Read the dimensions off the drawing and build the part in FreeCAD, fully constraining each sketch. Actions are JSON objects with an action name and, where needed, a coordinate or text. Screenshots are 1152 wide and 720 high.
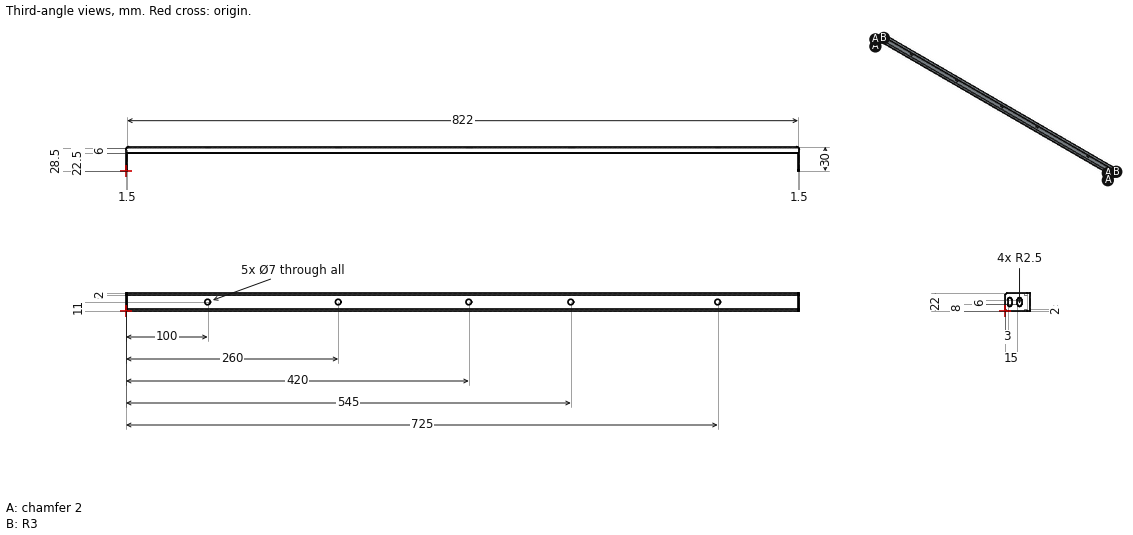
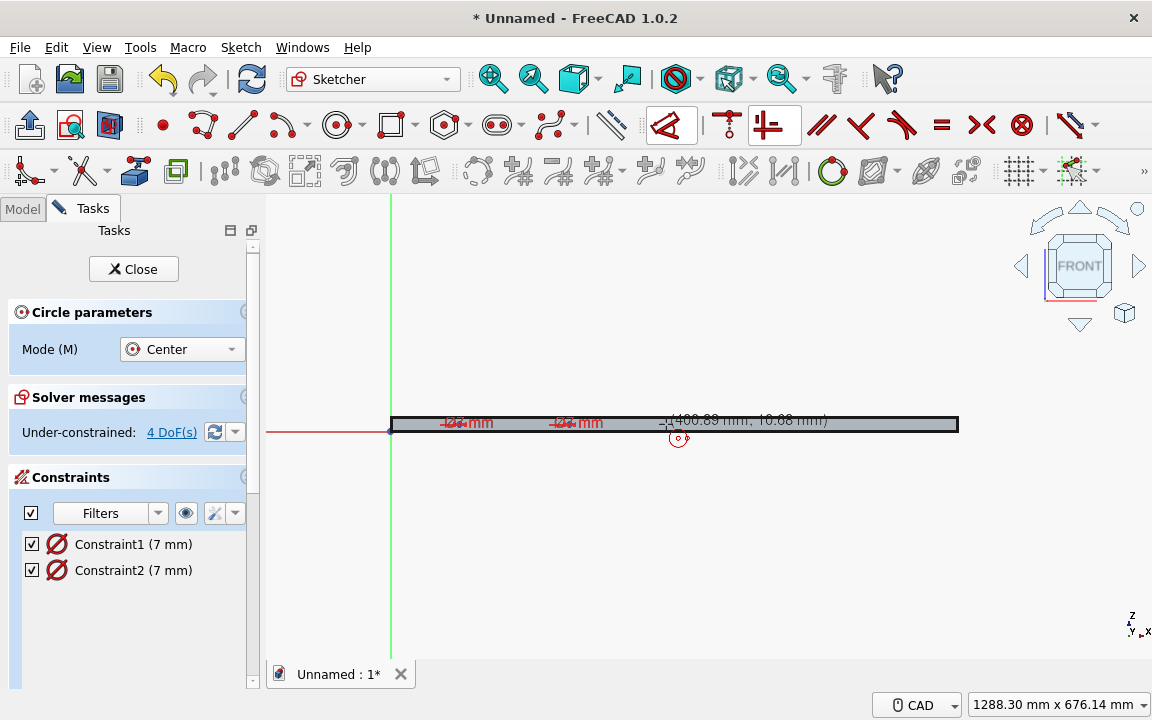
{"action": "scroll", "coordinate": [680, 424], "scroll_direction": "up", "scroll_amount": 4}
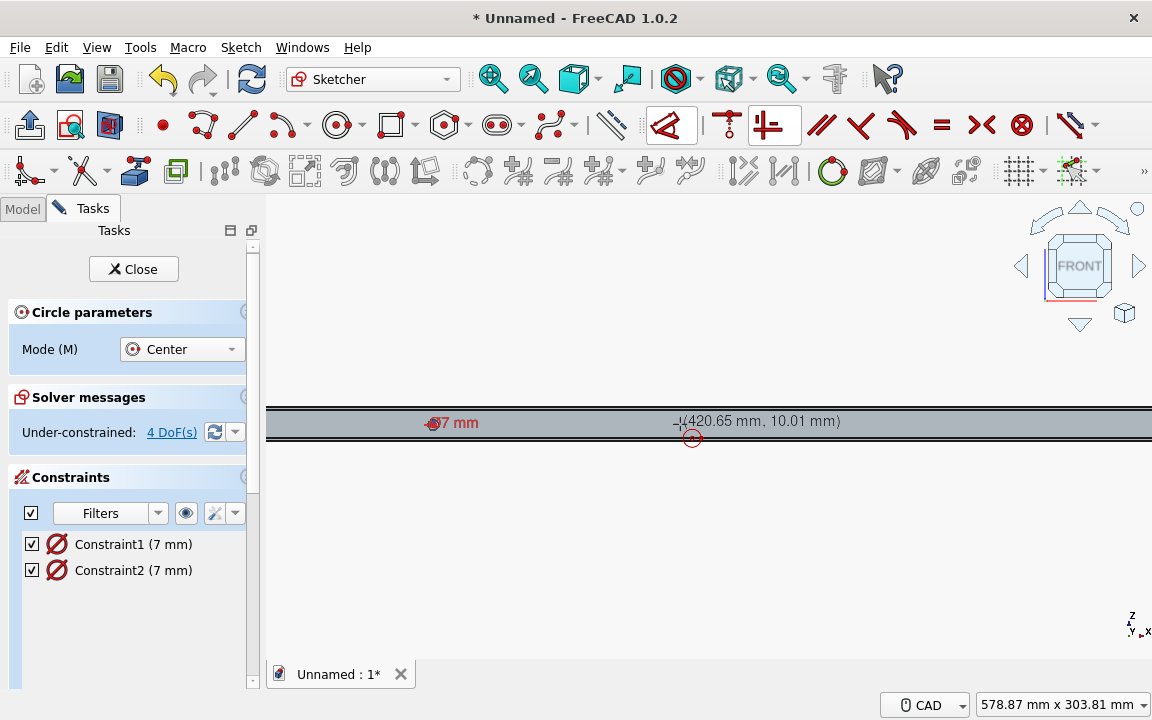
{"action": "left_click", "coordinate": [678, 424]}
{"action": "mouse_move", "coordinate": [682, 420]}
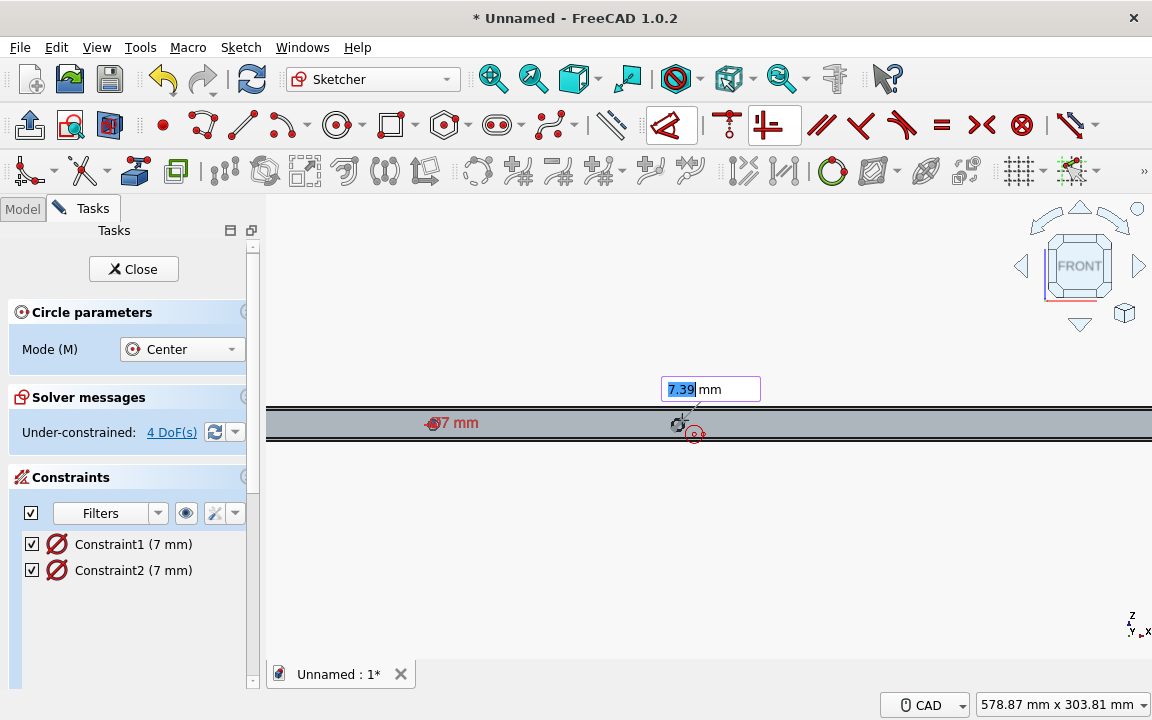
{"action": "type", "text": "7"}
{"action": "key", "text": "Return"}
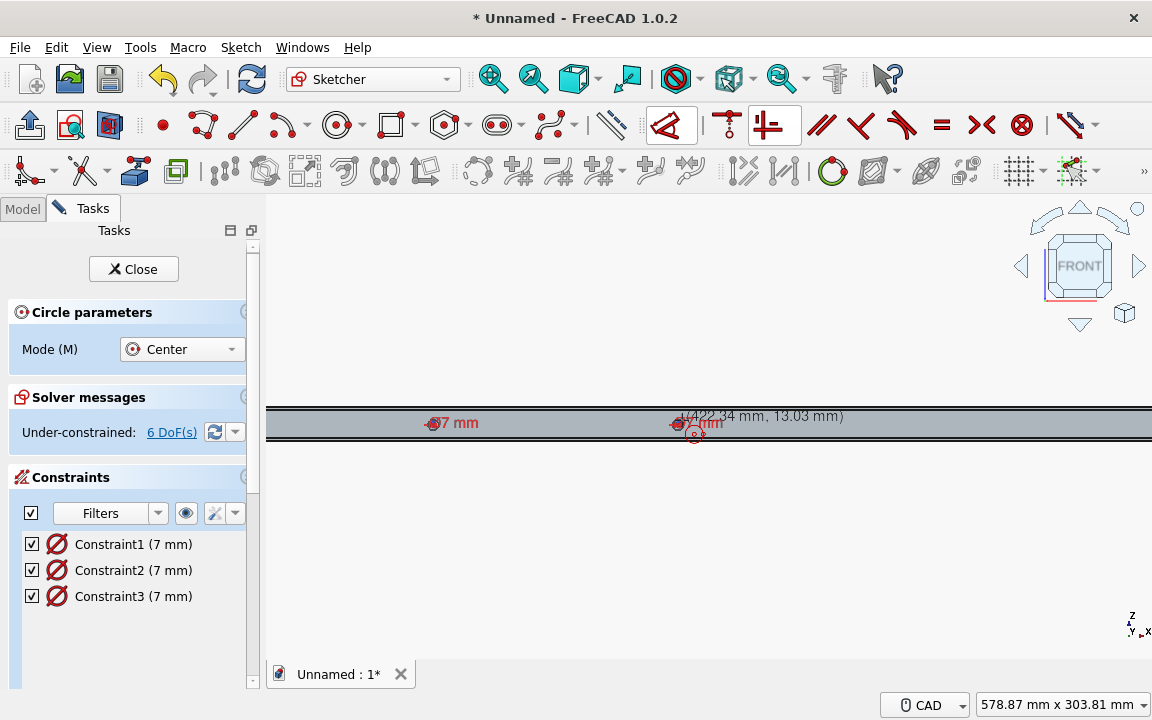
{"action": "scroll", "coordinate": [870, 424], "scroll_direction": "up", "scroll_amount": 8}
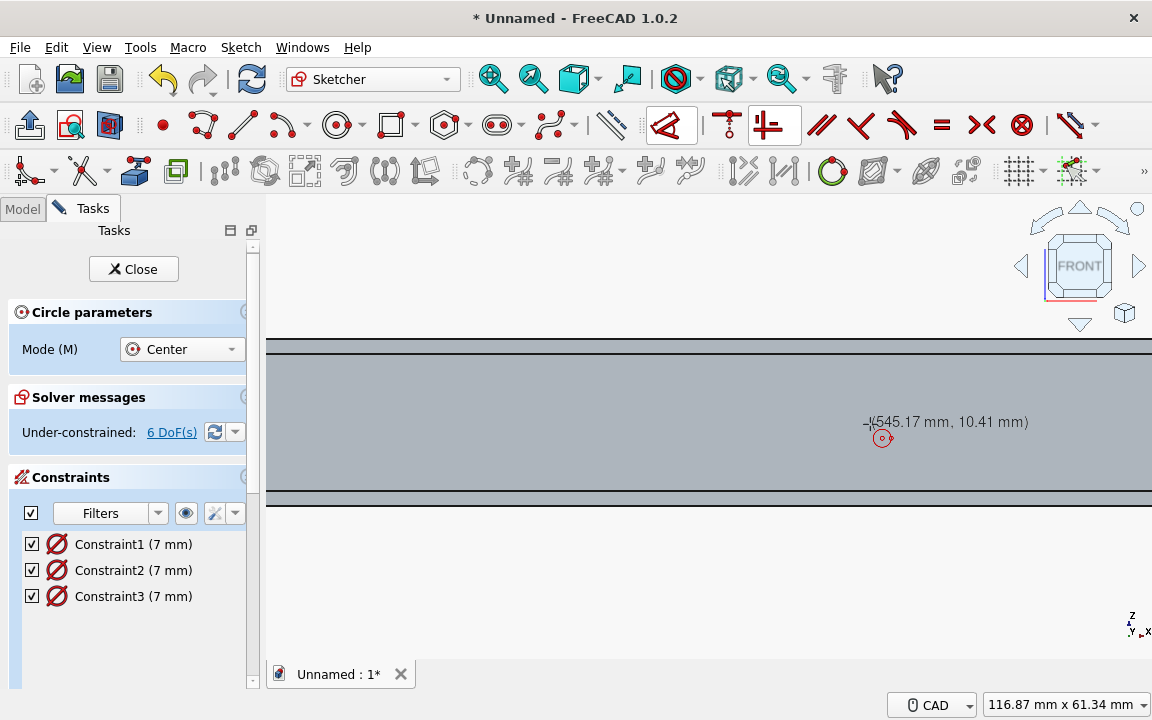
{"action": "scroll", "coordinate": [755, 424], "scroll_direction": "down", "scroll_amount": 12}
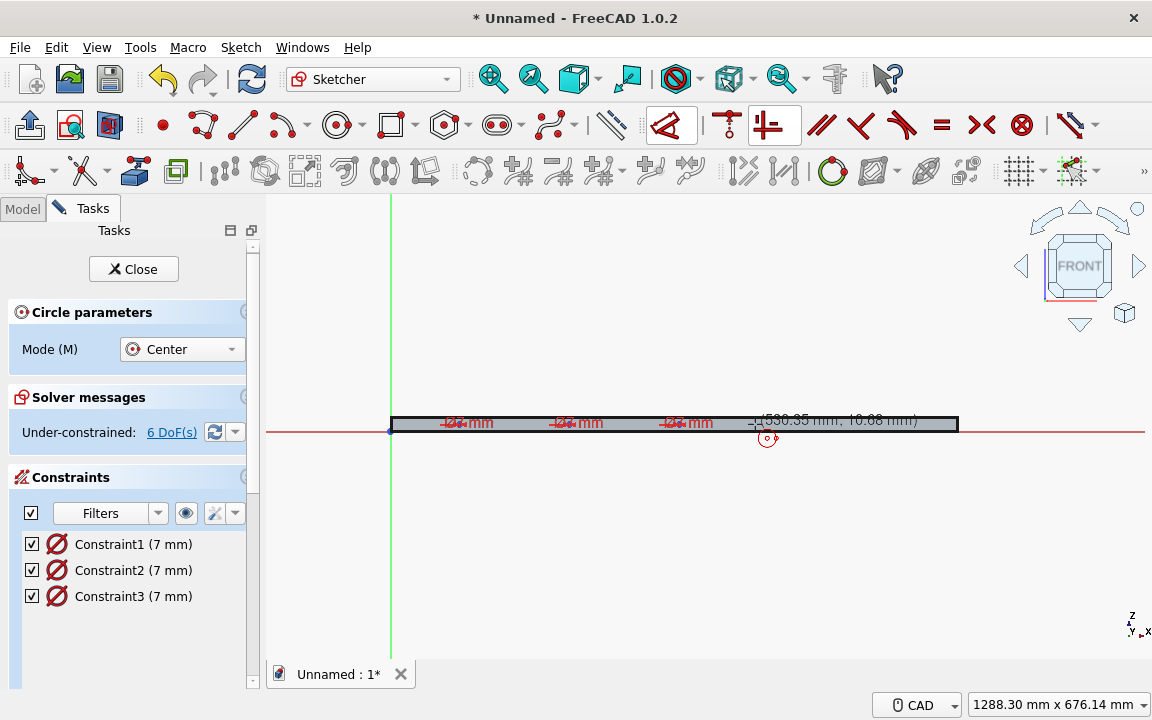
{"action": "scroll", "coordinate": [766, 424], "scroll_direction": "up", "scroll_amount": 4}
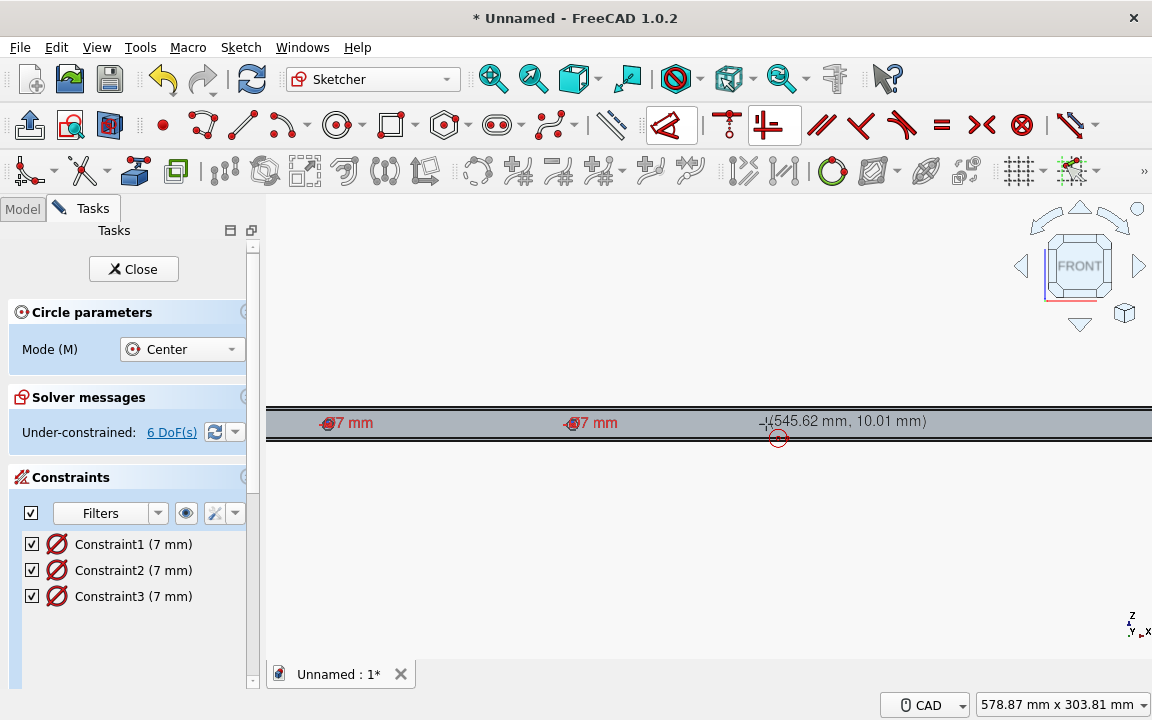
{"action": "left_click", "coordinate": [764, 424]}
{"action": "mouse_move", "coordinate": [768, 420]}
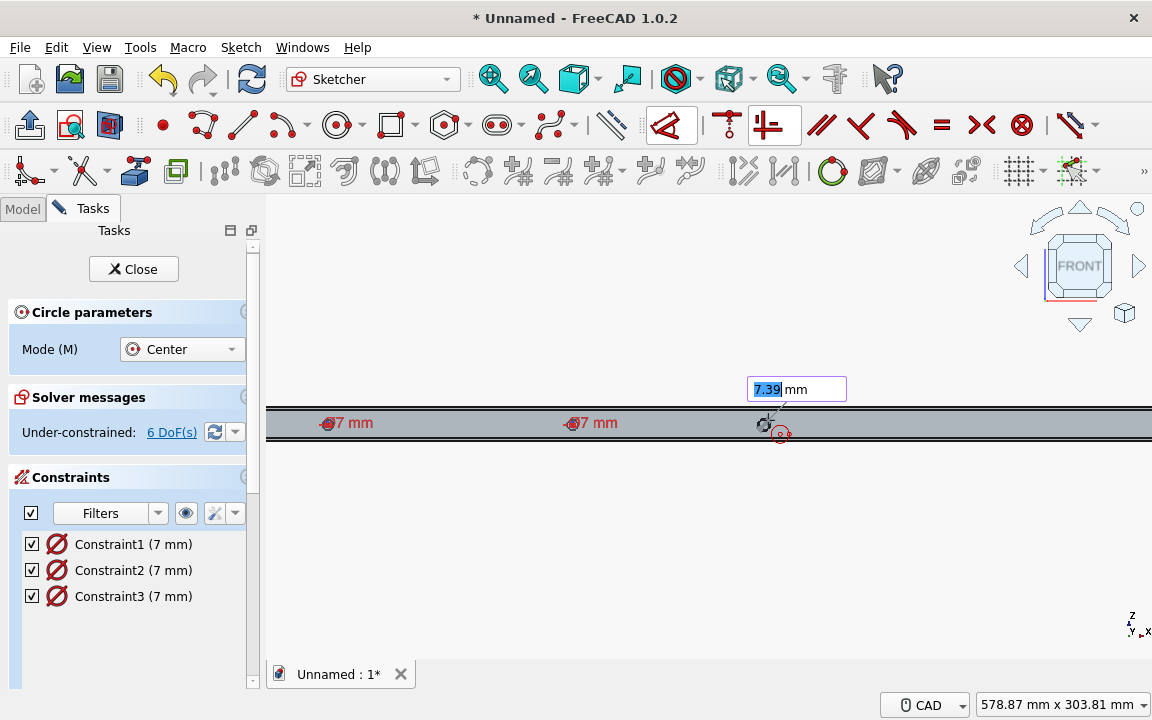
{"action": "type", "text": "7"}
{"action": "key", "text": "Return"}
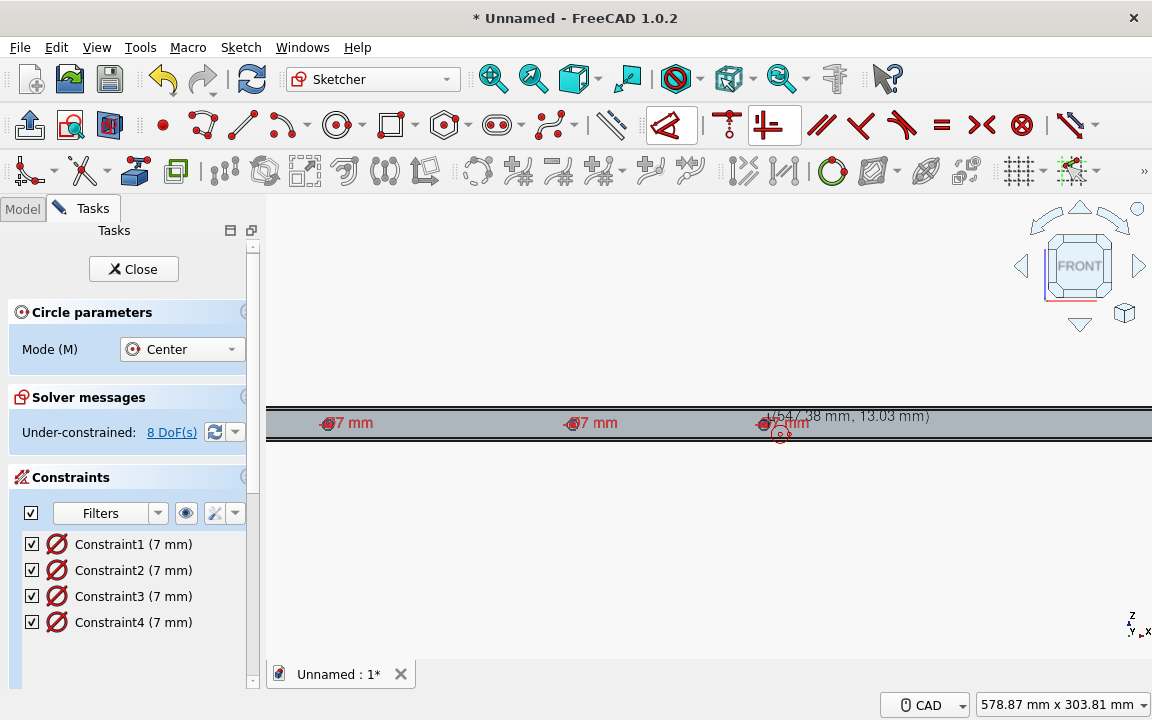
{"action": "scroll", "coordinate": [765, 424], "scroll_direction": "down", "scroll_amount": 4}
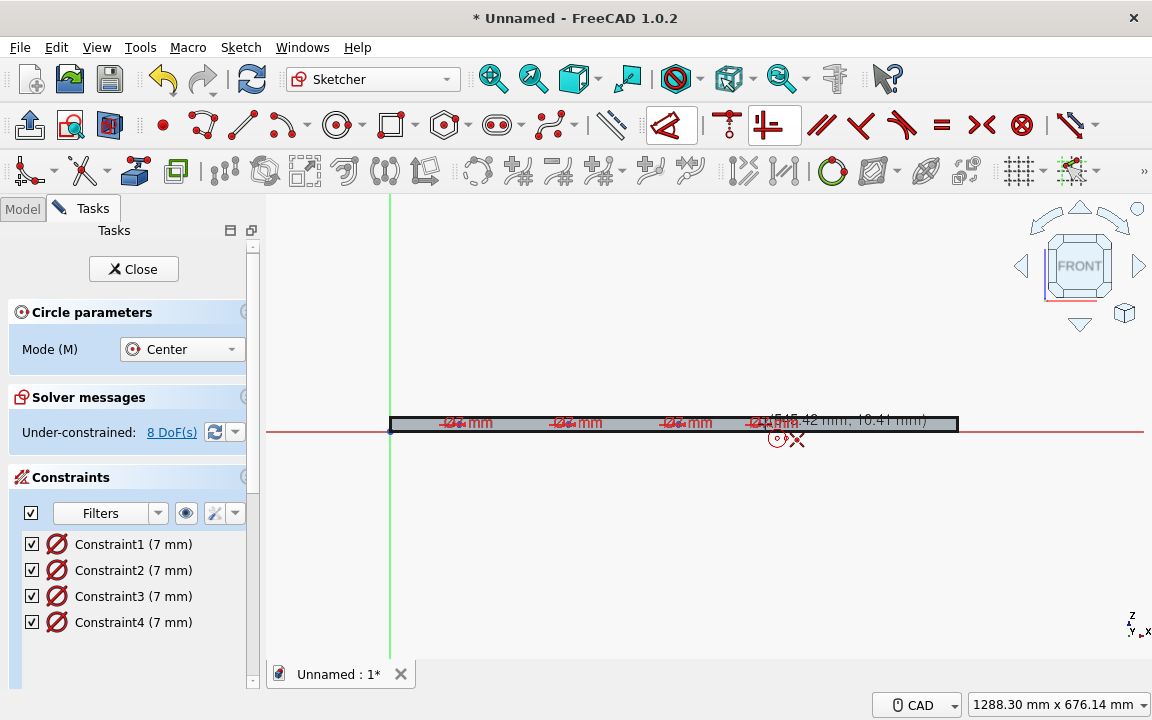
{"action": "scroll", "coordinate": [889, 424], "scroll_direction": "up", "scroll_amount": 12}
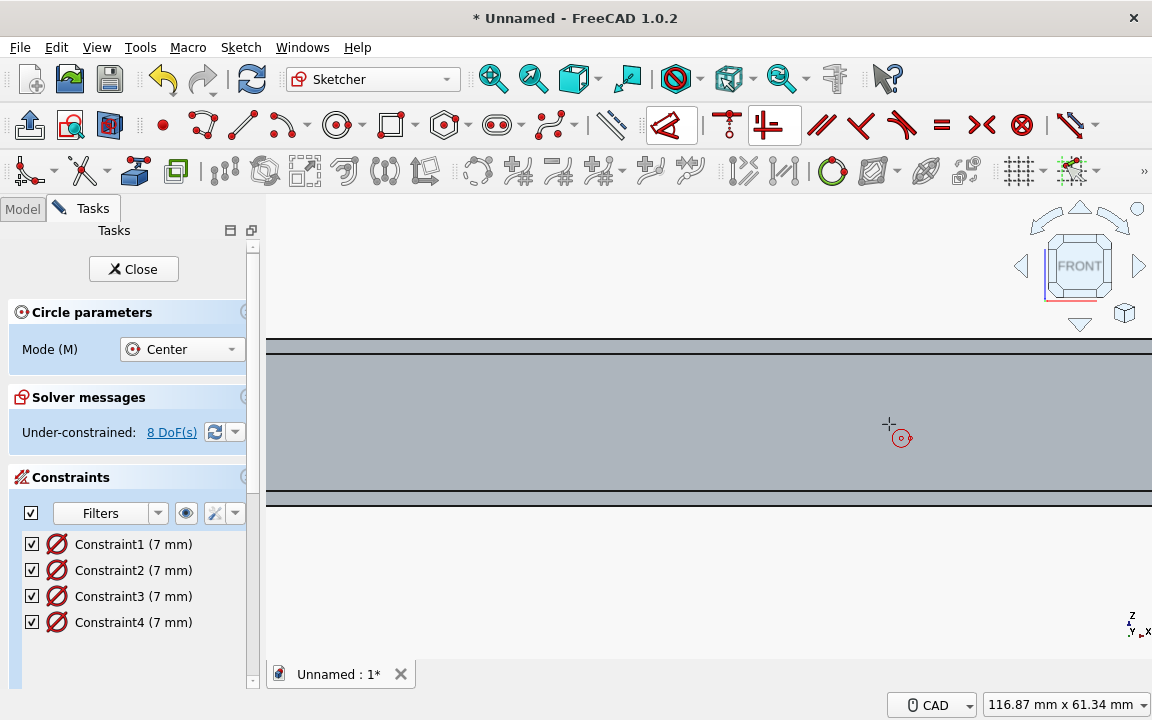
{"action": "scroll", "coordinate": [889, 424], "scroll_direction": "down", "scroll_amount": 12}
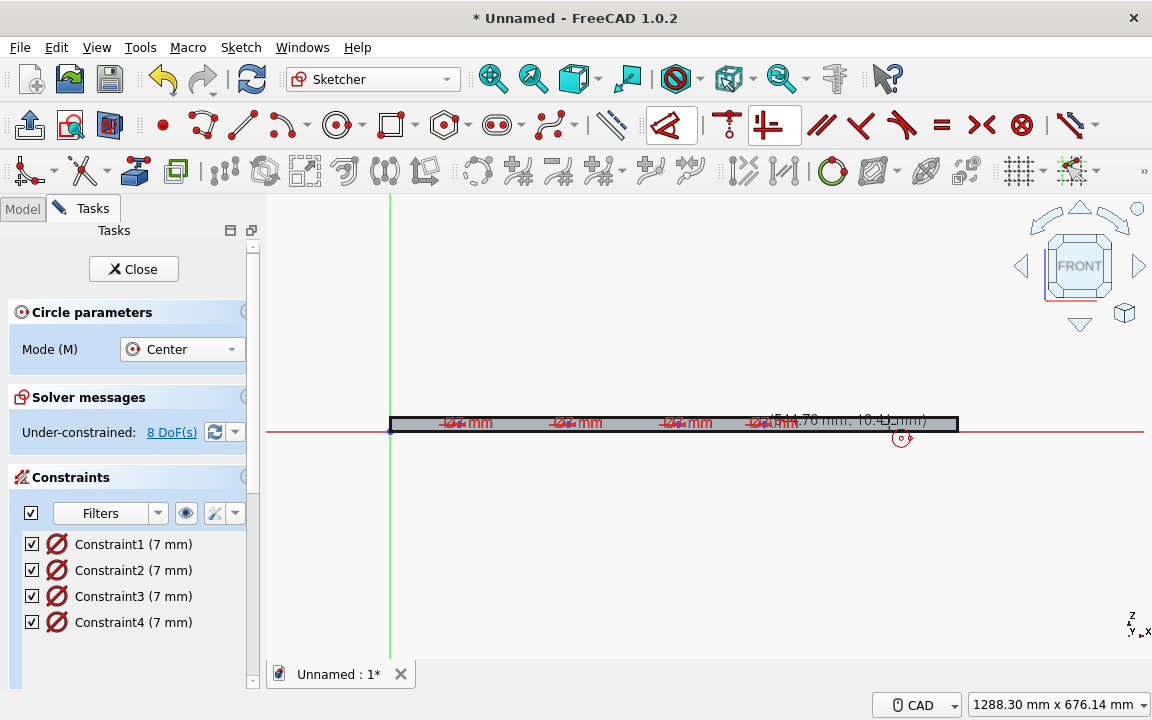
{"action": "scroll", "coordinate": [889, 424], "scroll_direction": "up", "scroll_amount": 4}